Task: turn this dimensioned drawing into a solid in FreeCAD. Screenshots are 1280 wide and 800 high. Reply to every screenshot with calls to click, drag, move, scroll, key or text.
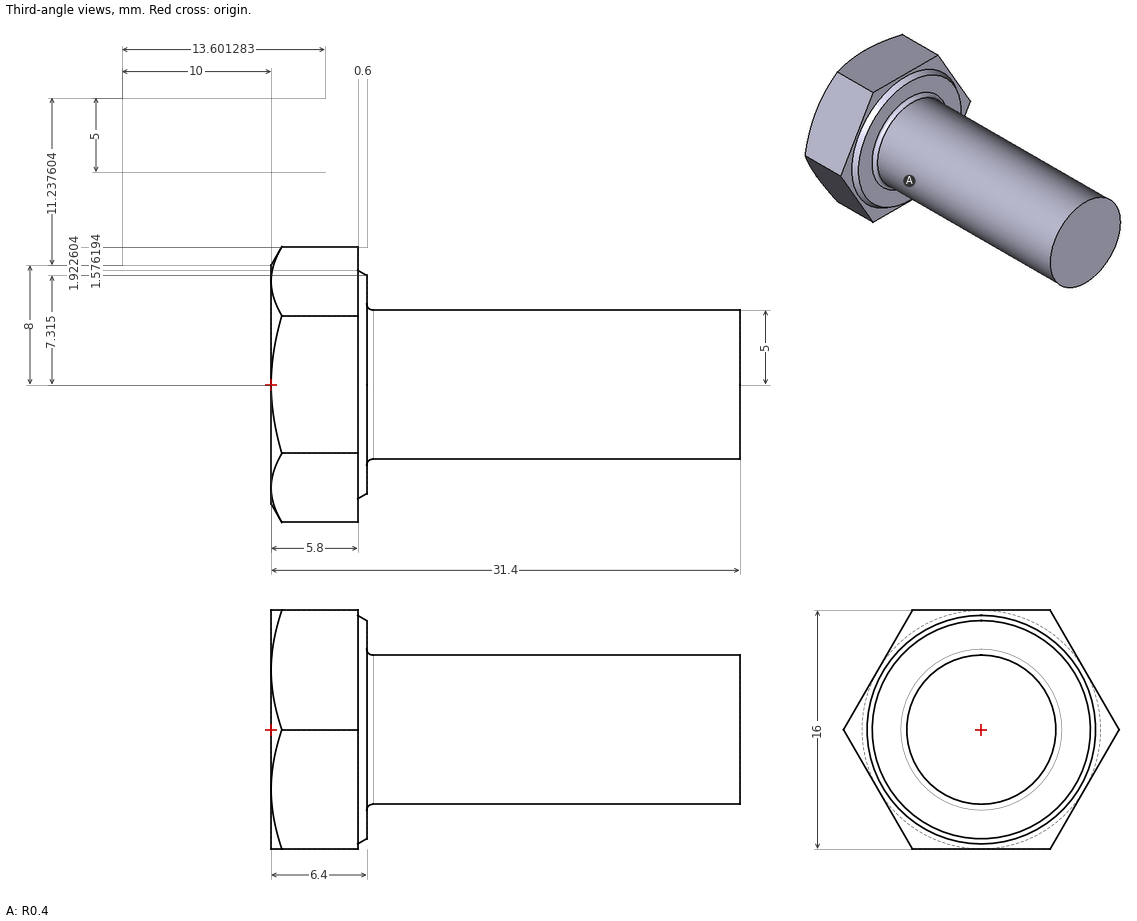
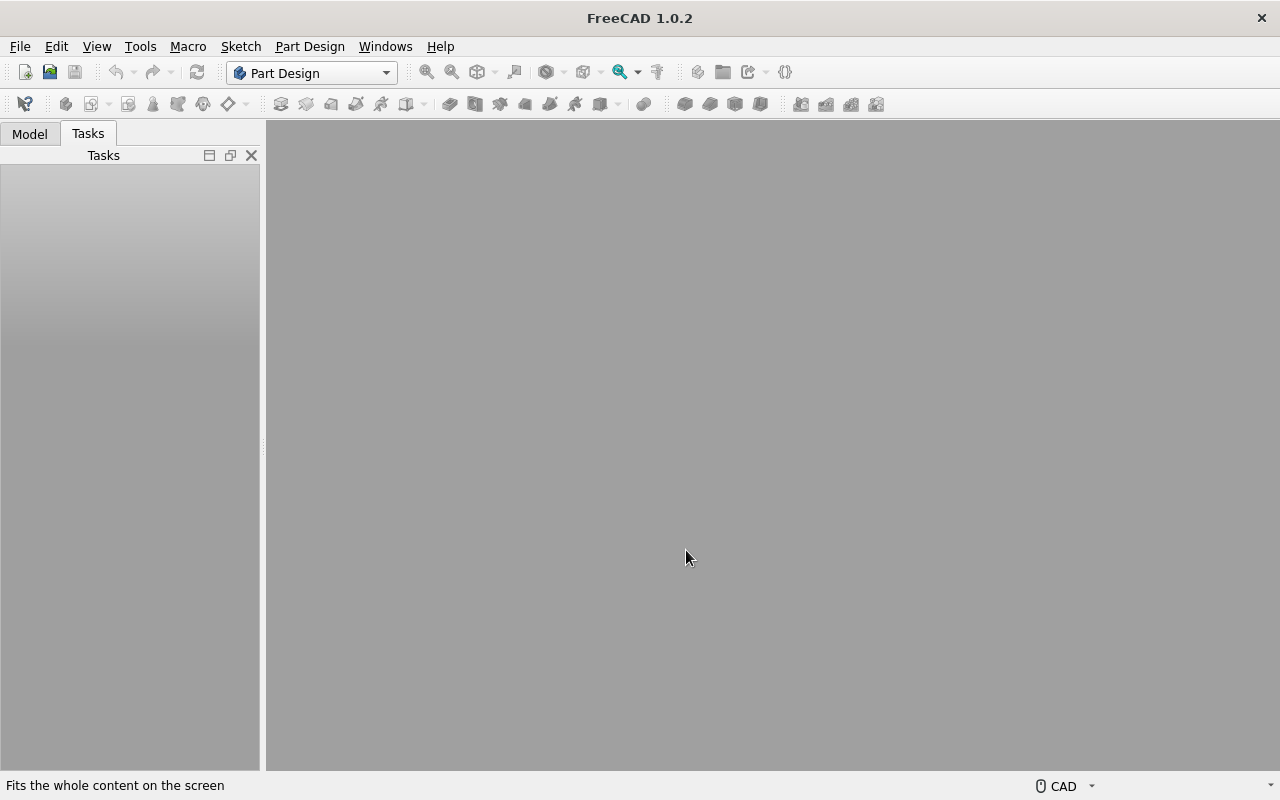
click(25, 72)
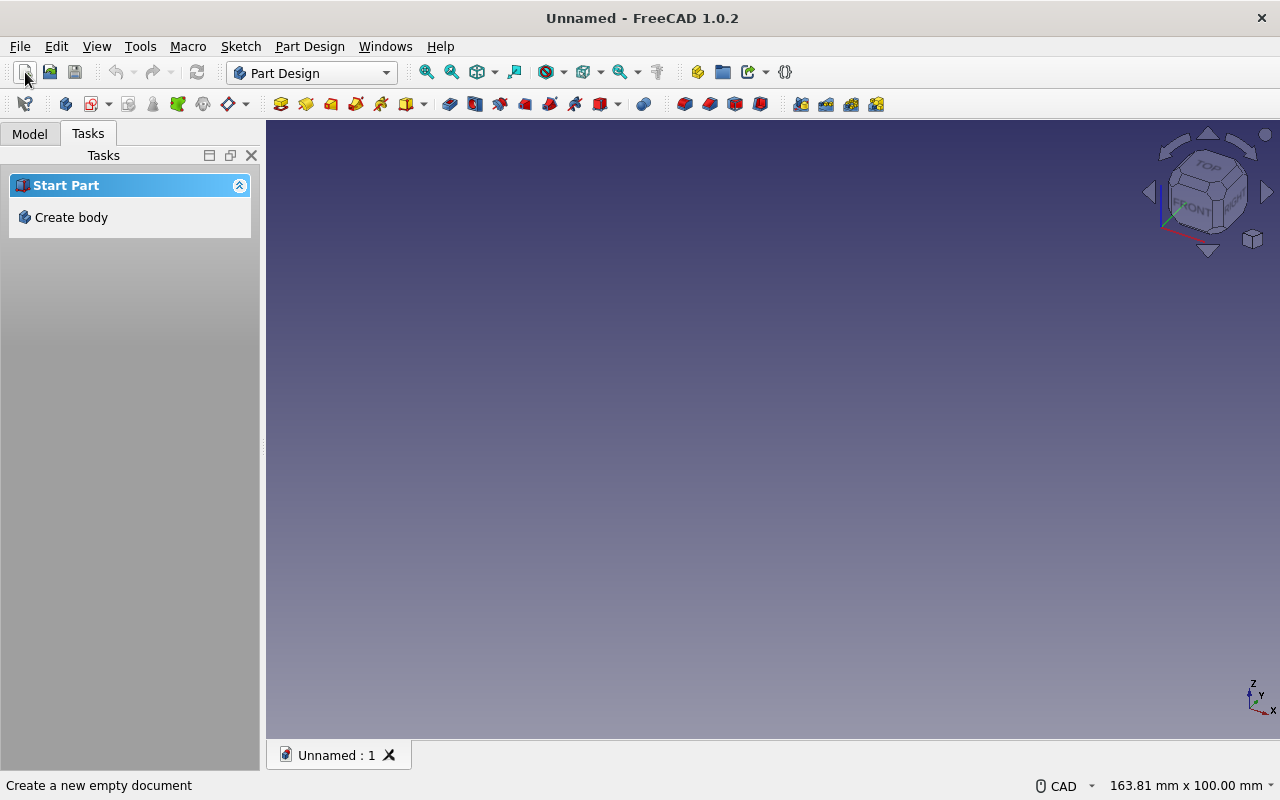
click(90, 104)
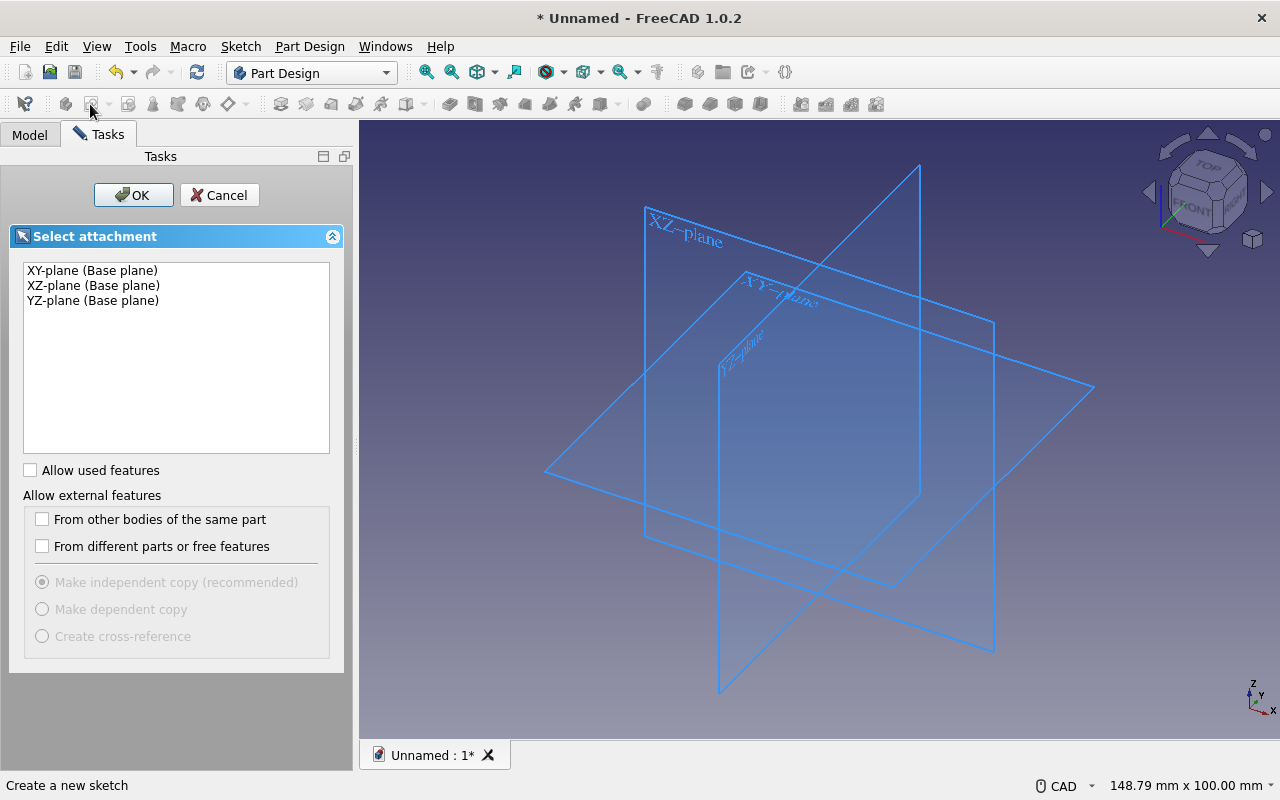
click(84, 300)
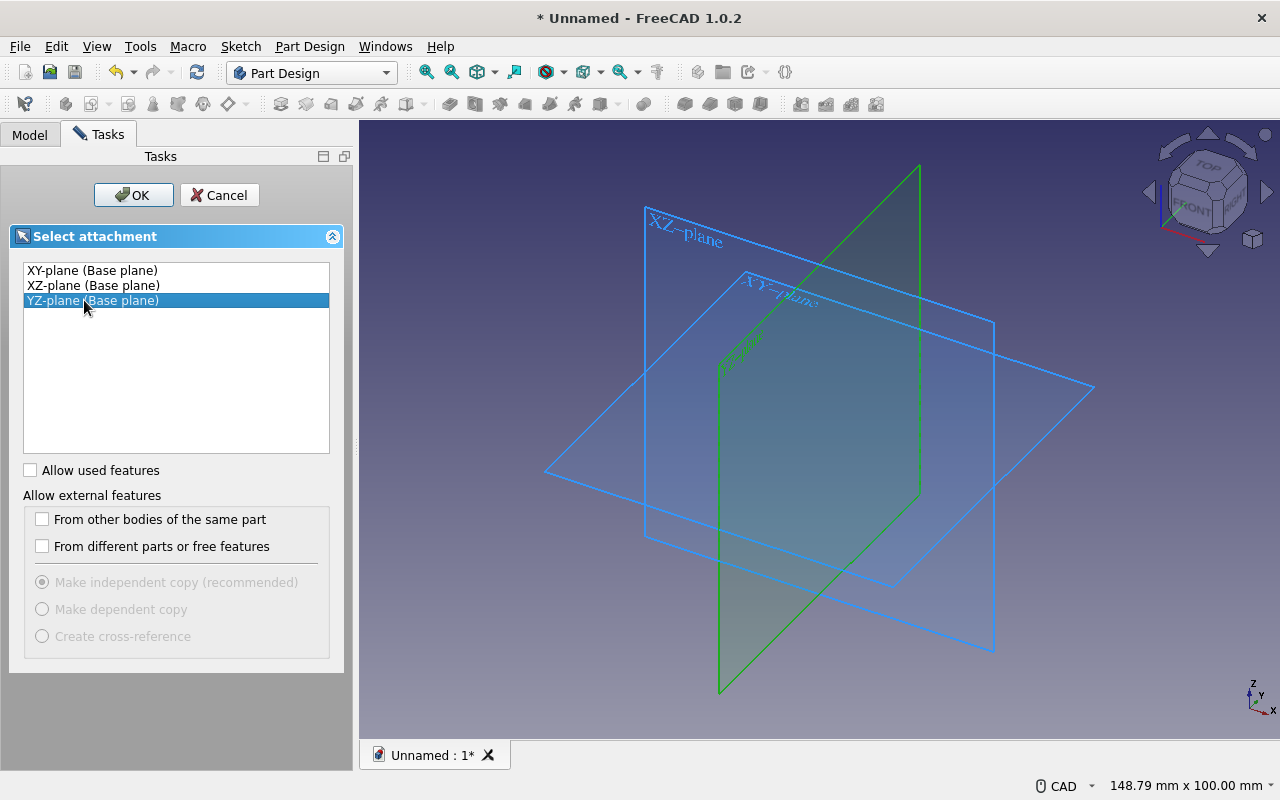
click(134, 195)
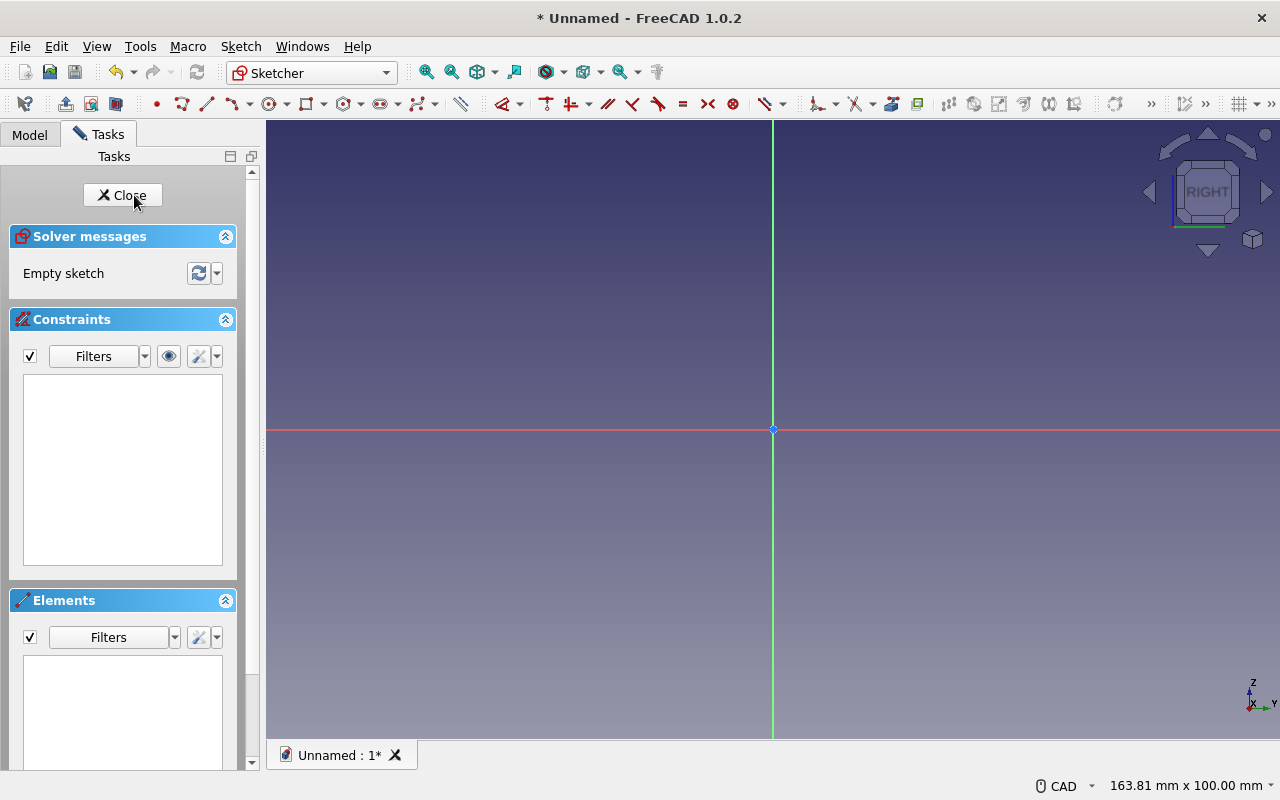
scroll(795, 430, up, 7)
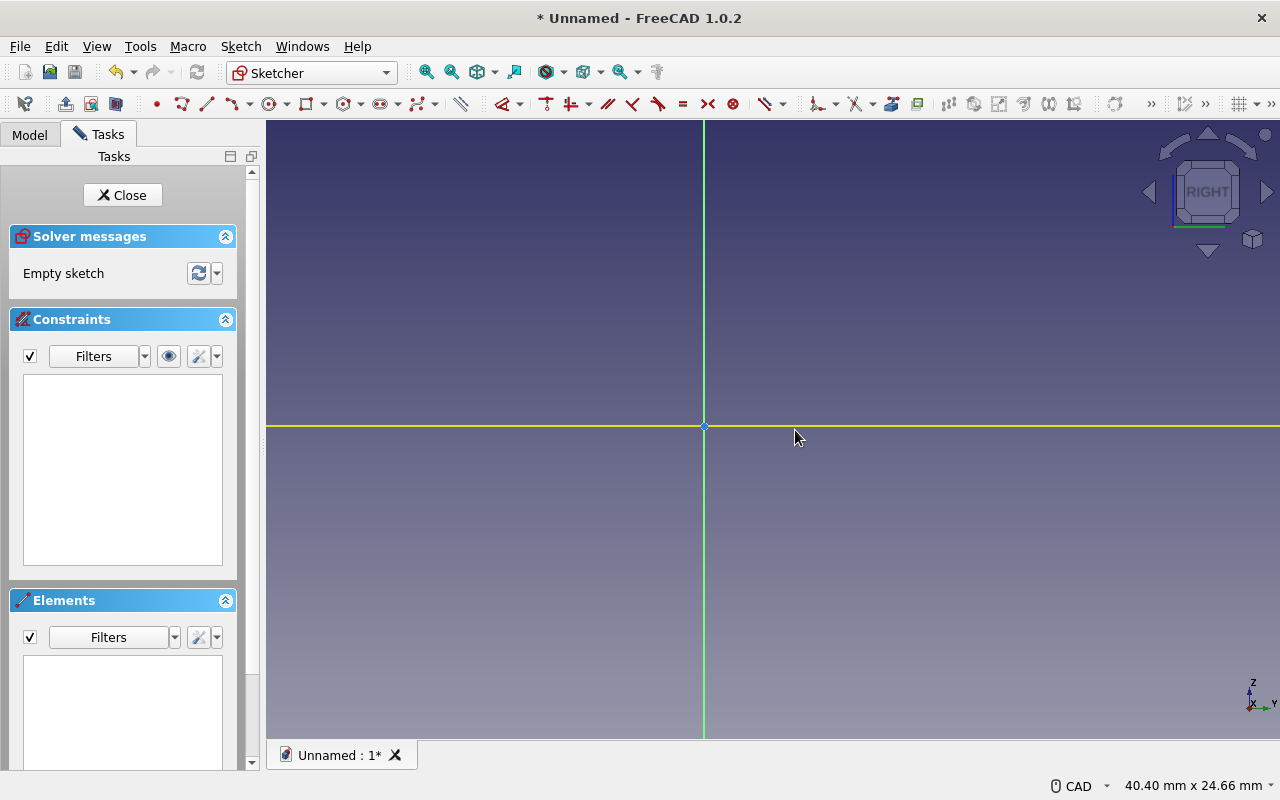
click(342, 104)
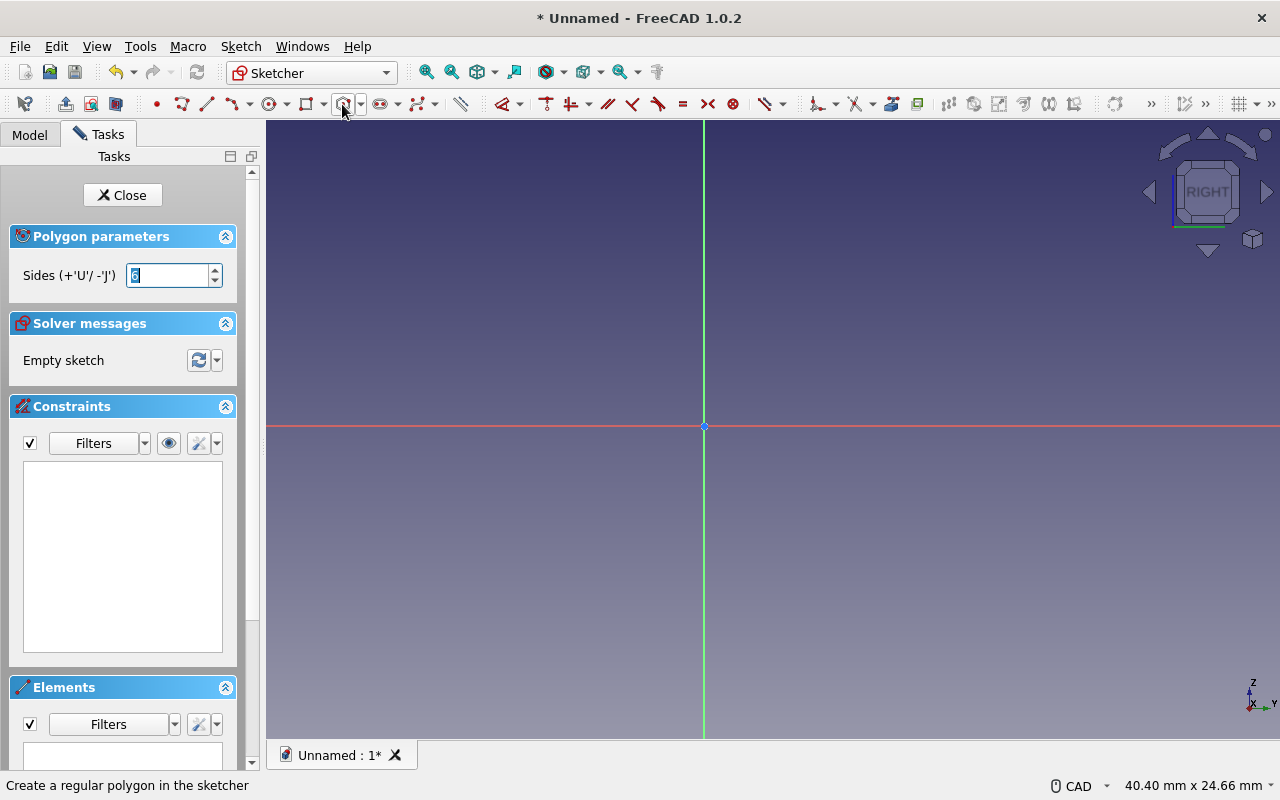
click(704, 426)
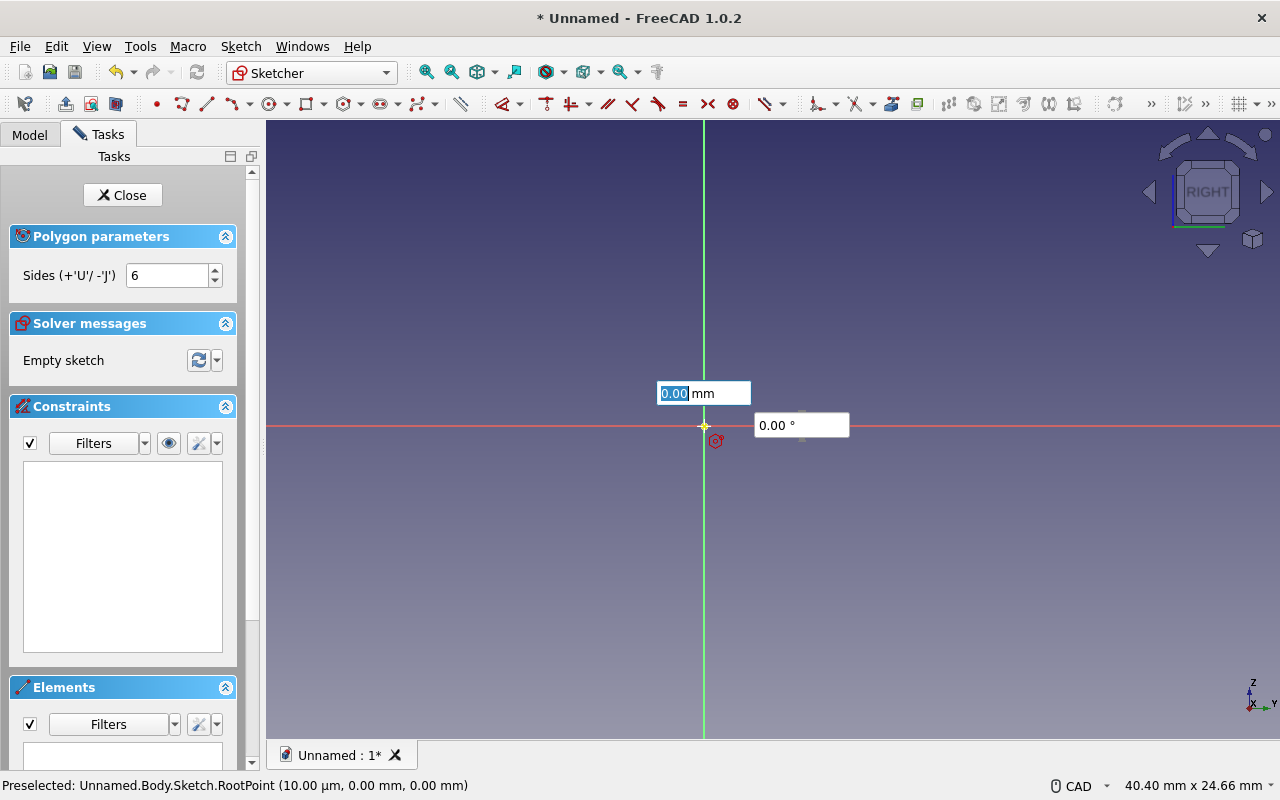
click(936, 426)
right_click(936, 426)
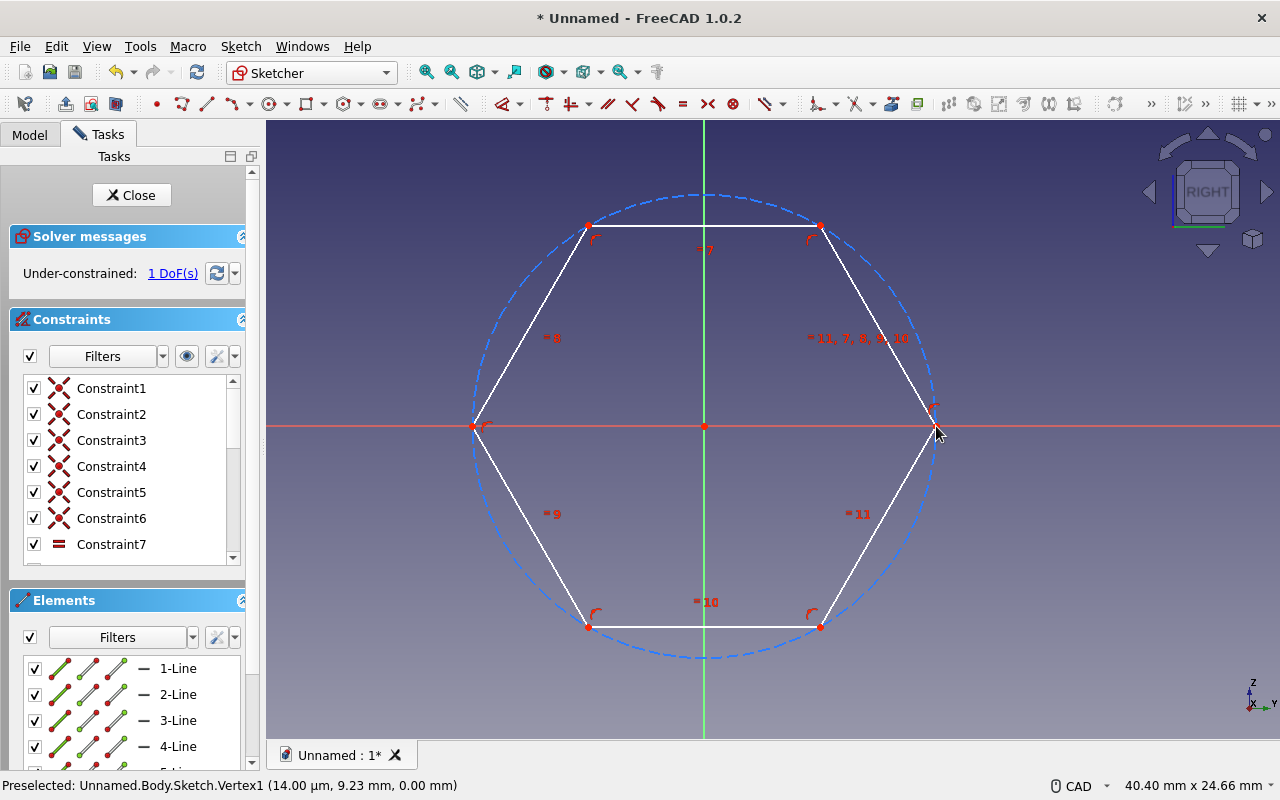
click(588, 627)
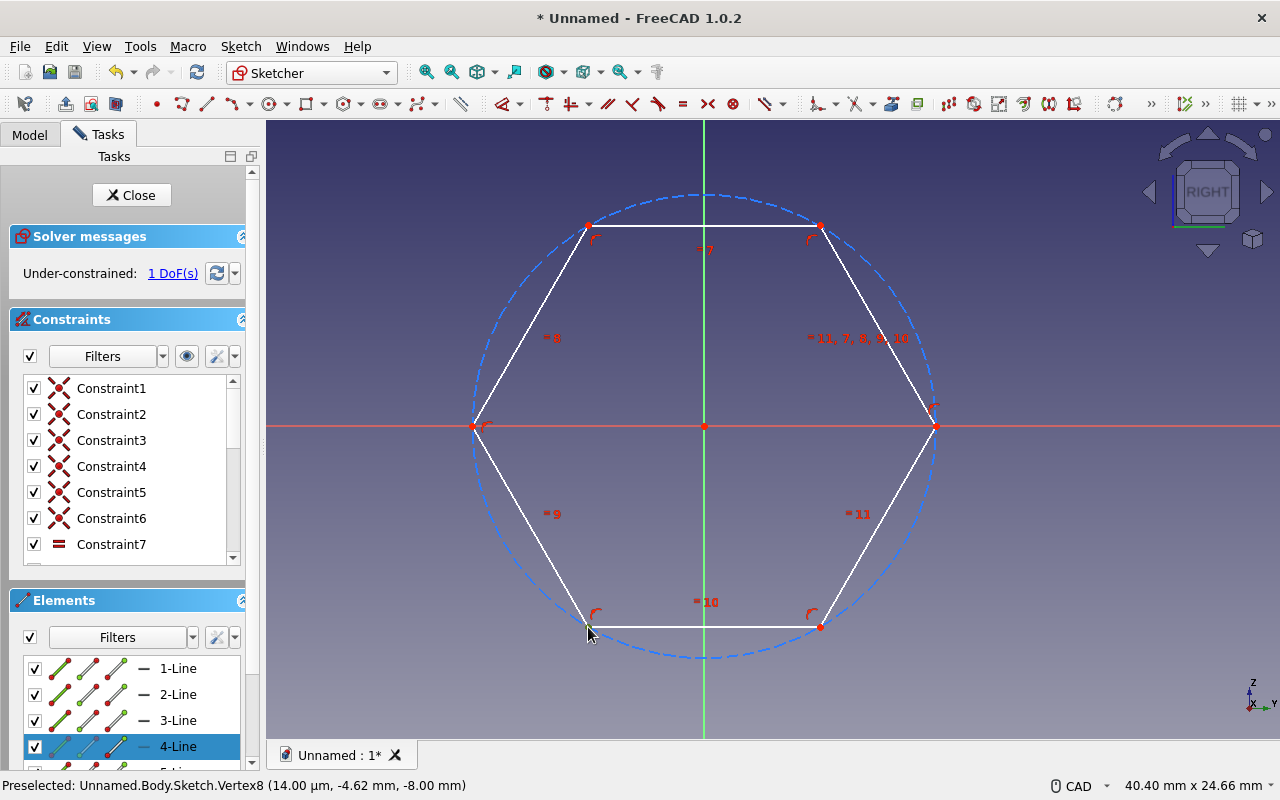
click(820, 226)